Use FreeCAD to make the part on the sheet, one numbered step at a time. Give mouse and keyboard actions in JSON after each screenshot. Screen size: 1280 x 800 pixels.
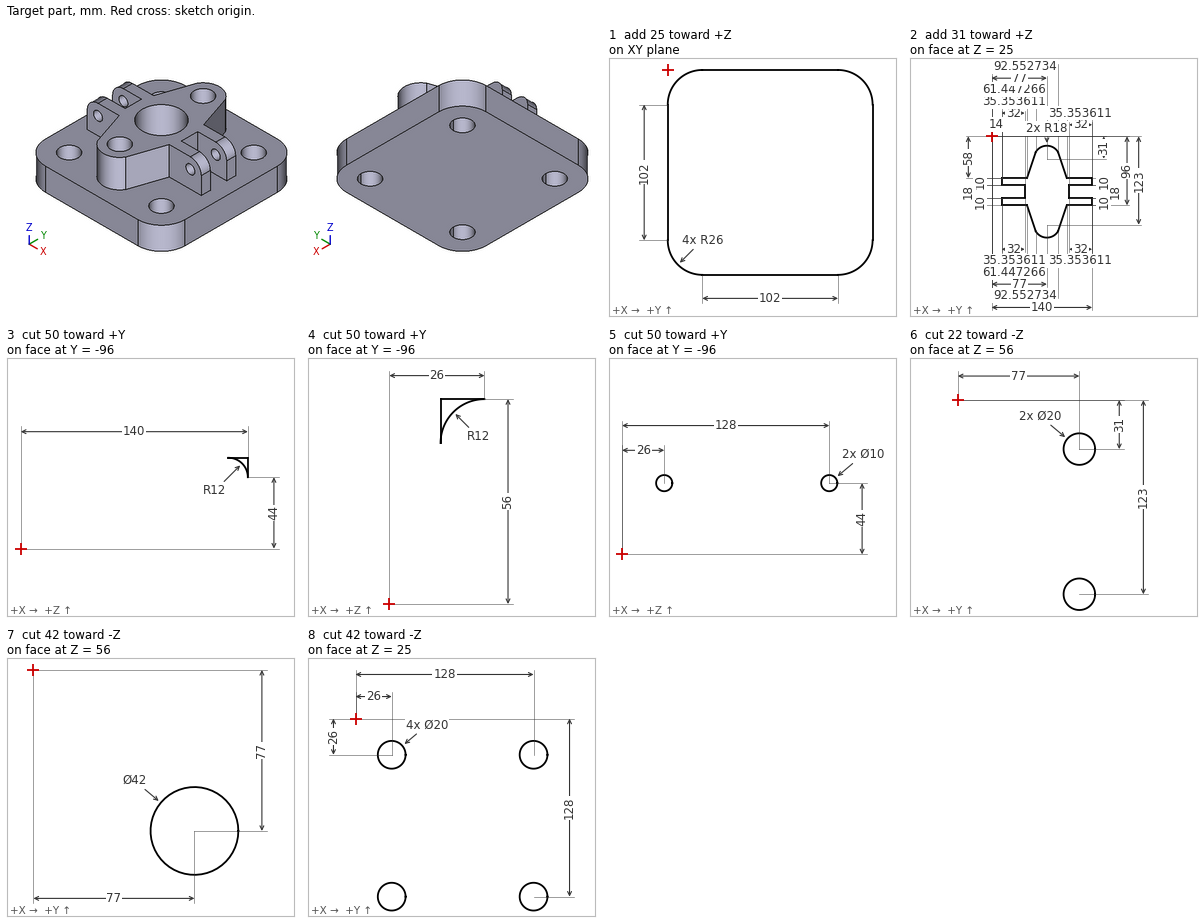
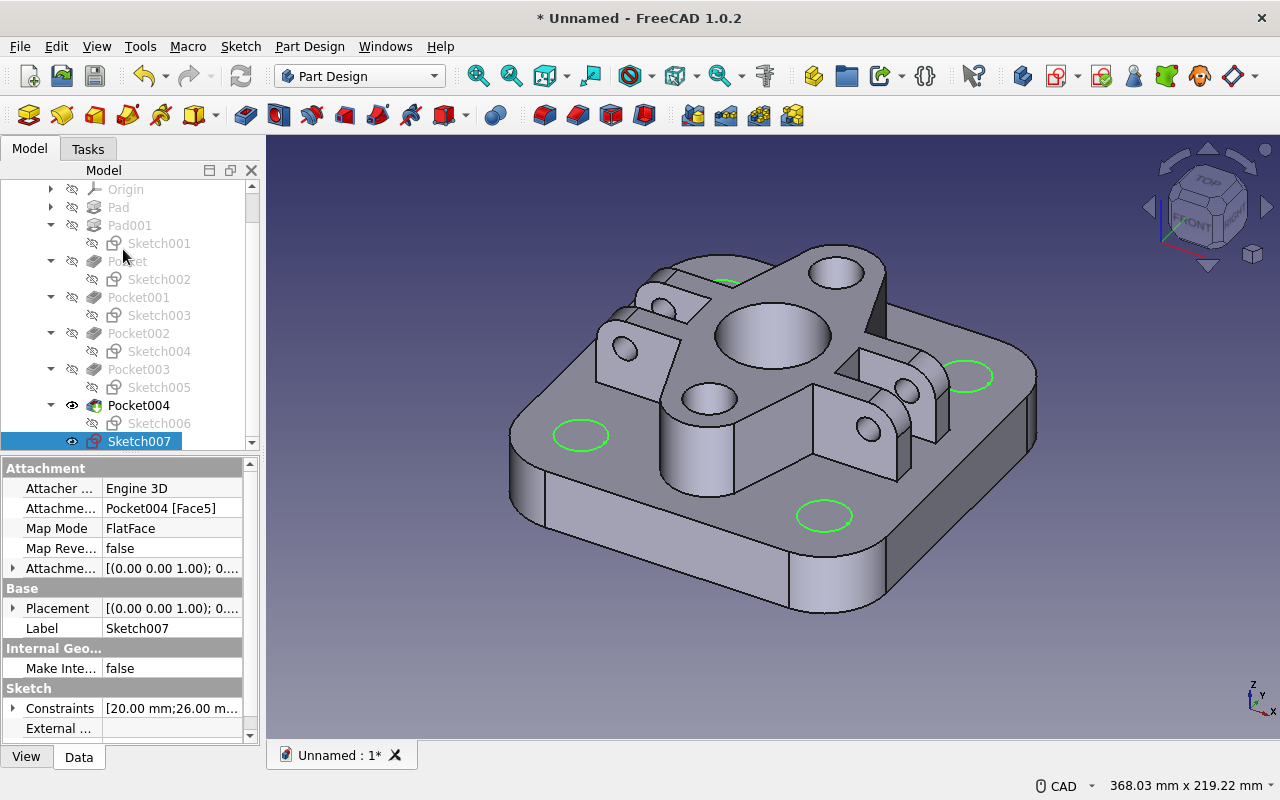
{"action": "left_click", "coordinate": [246, 116]}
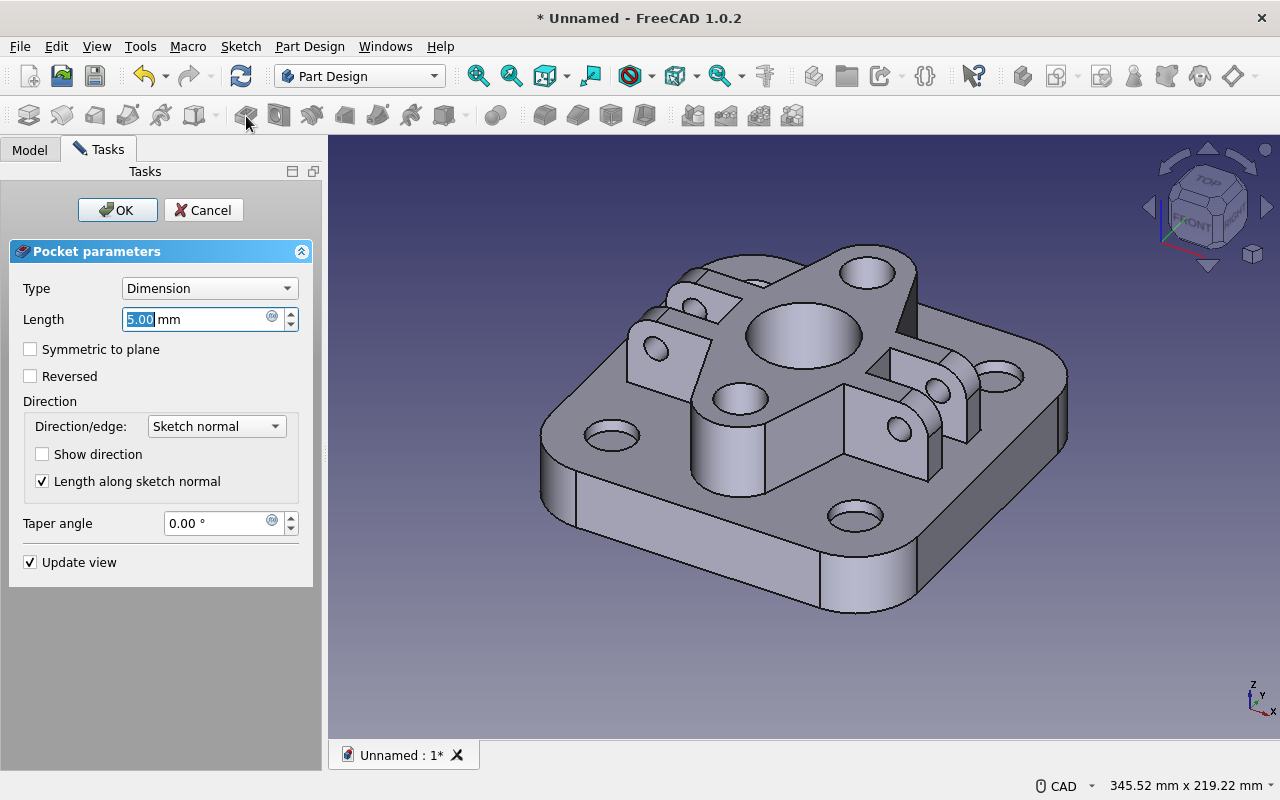
{"action": "type", "text": "42"}
{"action": "key", "text": "Tab"}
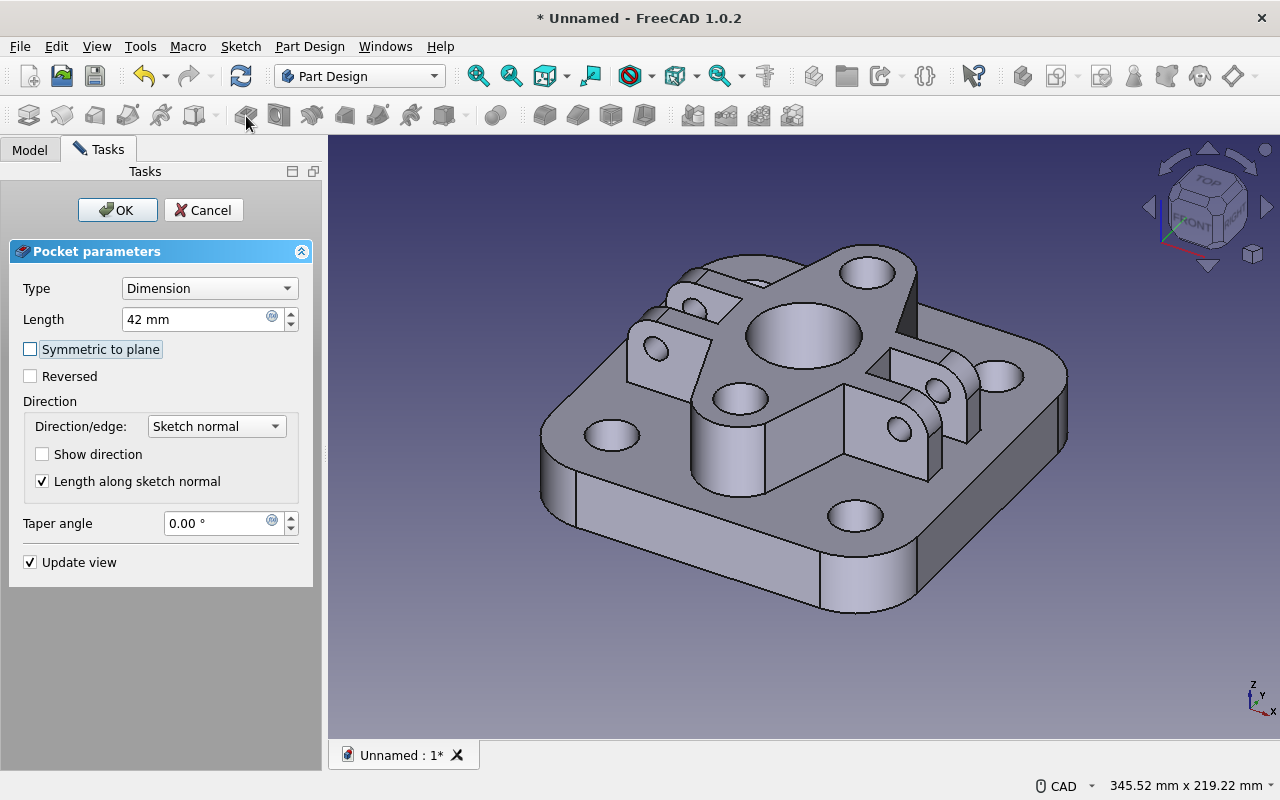
{"action": "left_click", "coordinate": [118, 210]}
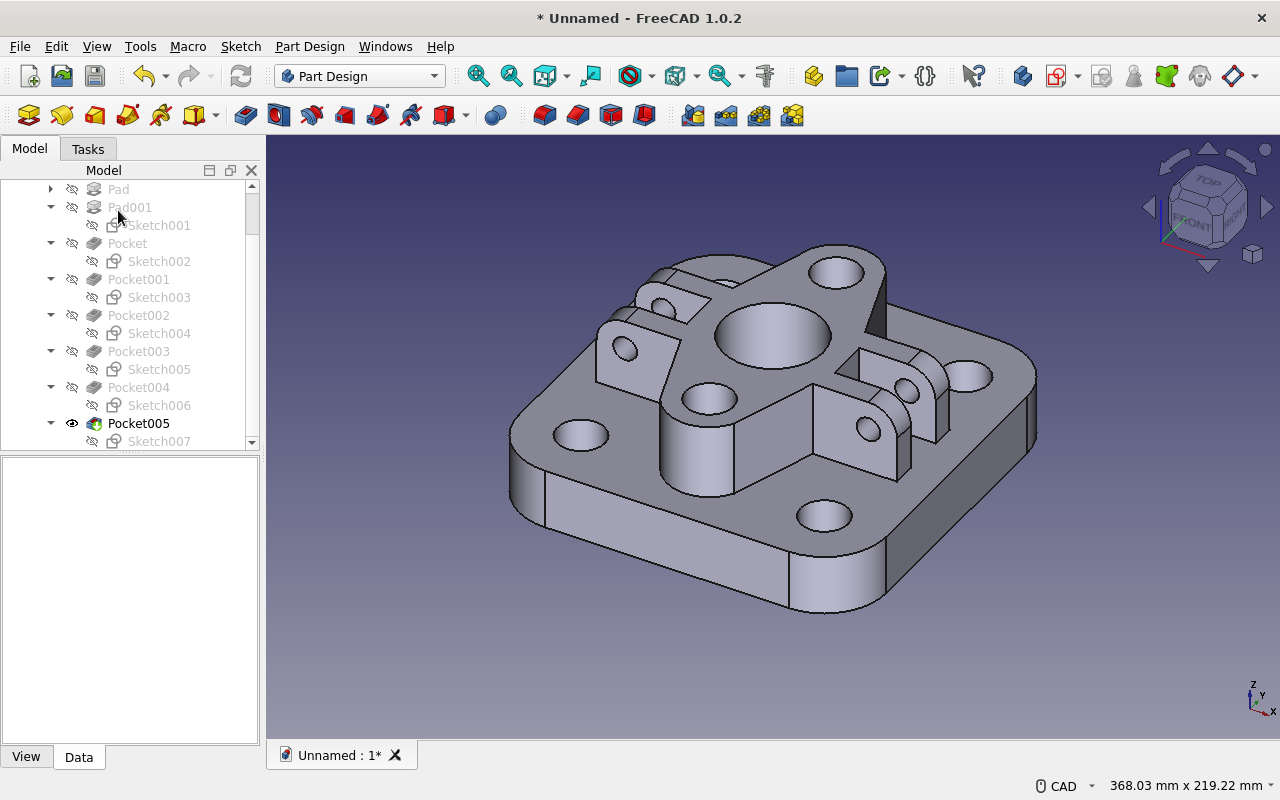
{"action": "key", "text": "0"}